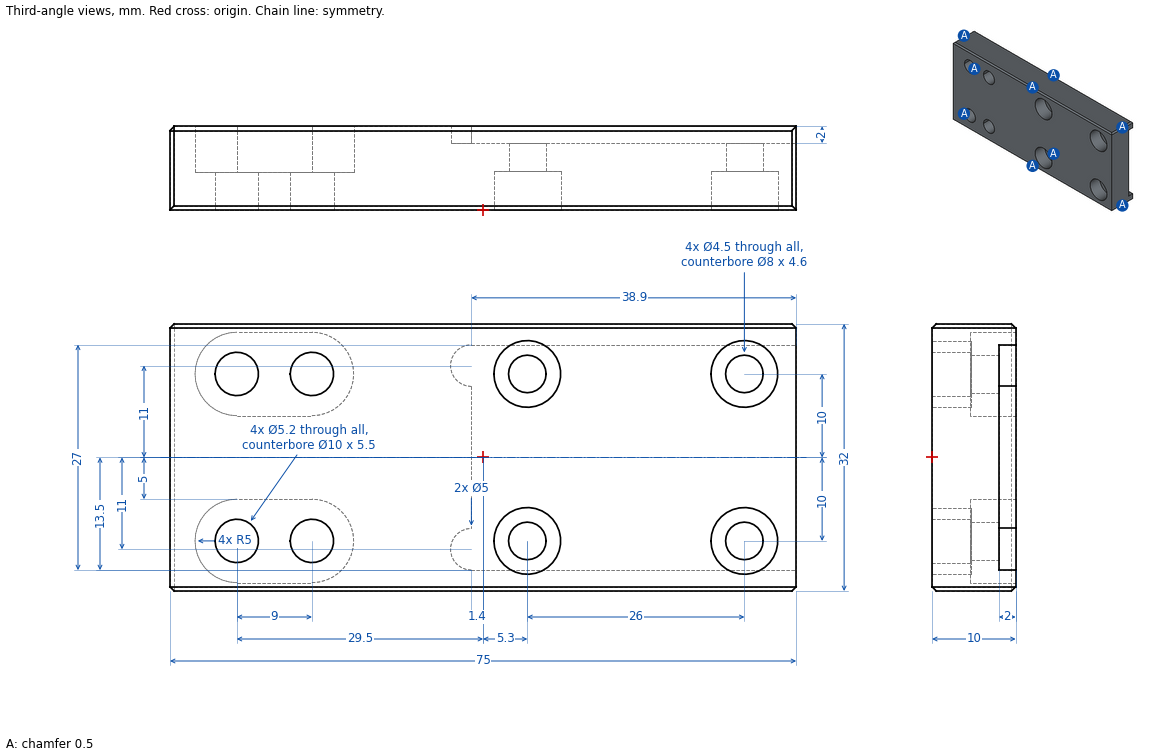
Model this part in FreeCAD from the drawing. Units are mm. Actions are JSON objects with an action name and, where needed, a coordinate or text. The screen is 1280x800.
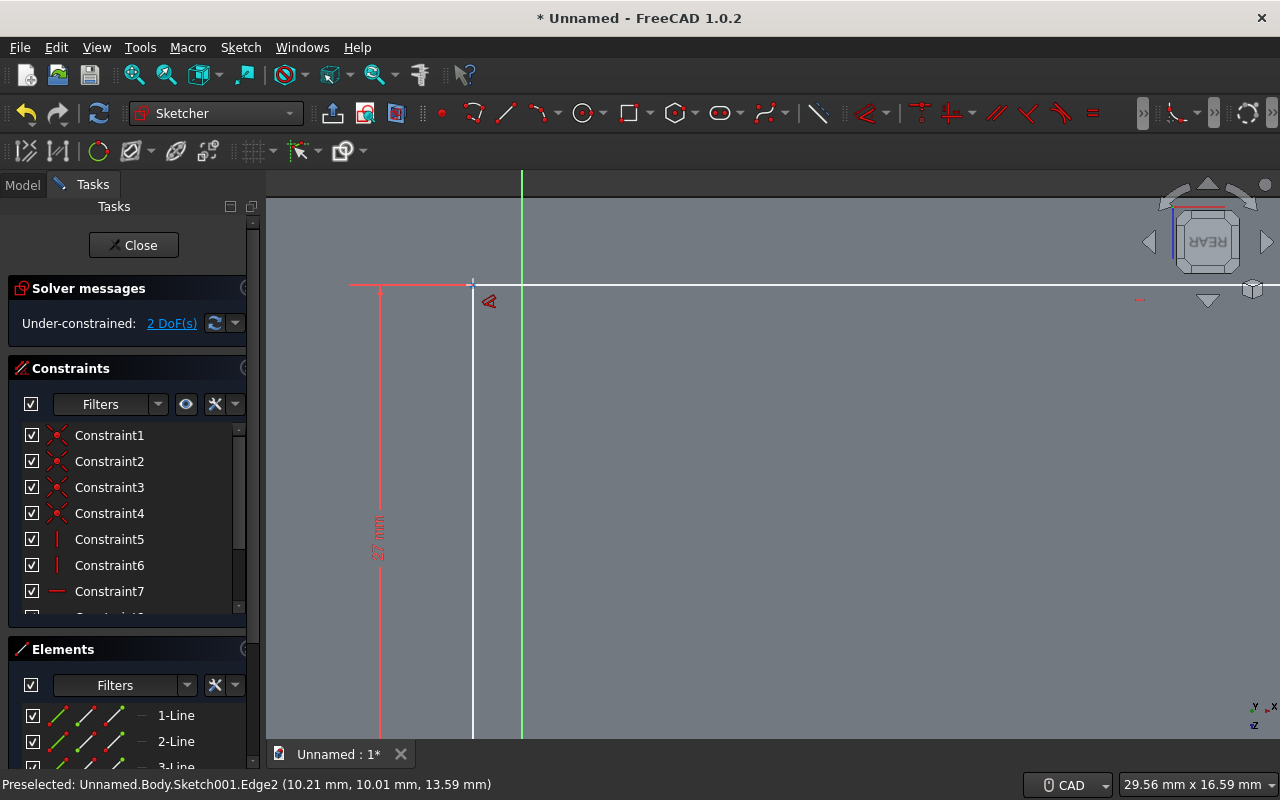
{"action": "left_click", "coordinate": [473, 285]}
{"action": "left_click", "coordinate": [497, 251]}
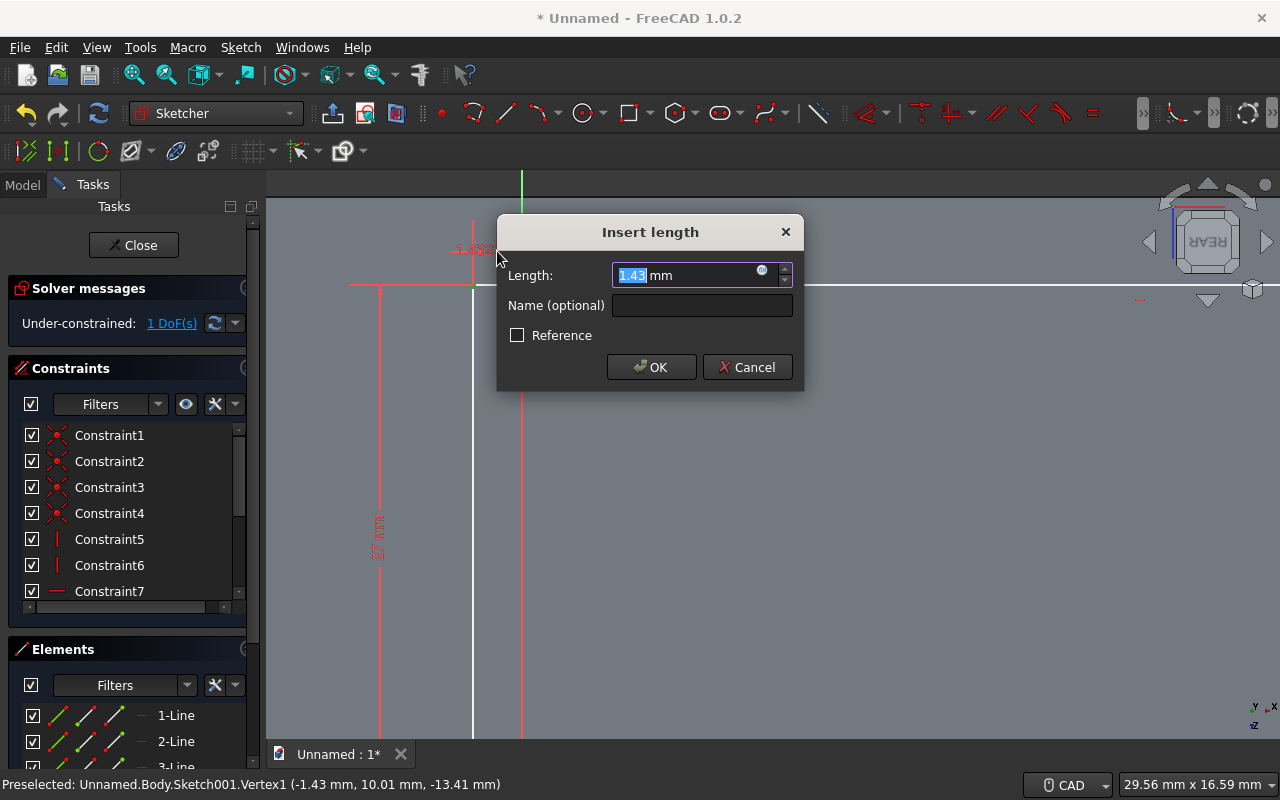
{"action": "type", "text": "1.4"}
{"action": "key", "text": "Return"}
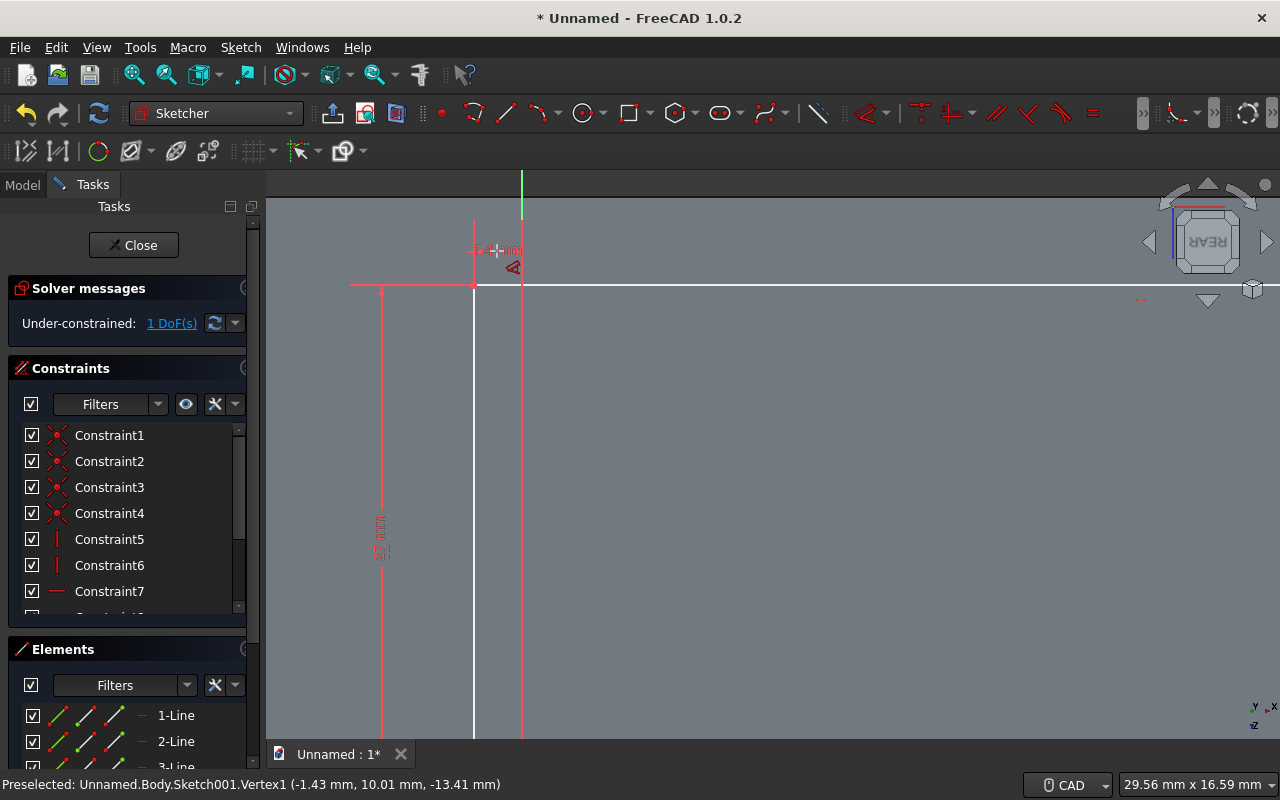
{"action": "left_click", "coordinate": [474, 285]}
{"action": "left_click", "coordinate": [440, 498]}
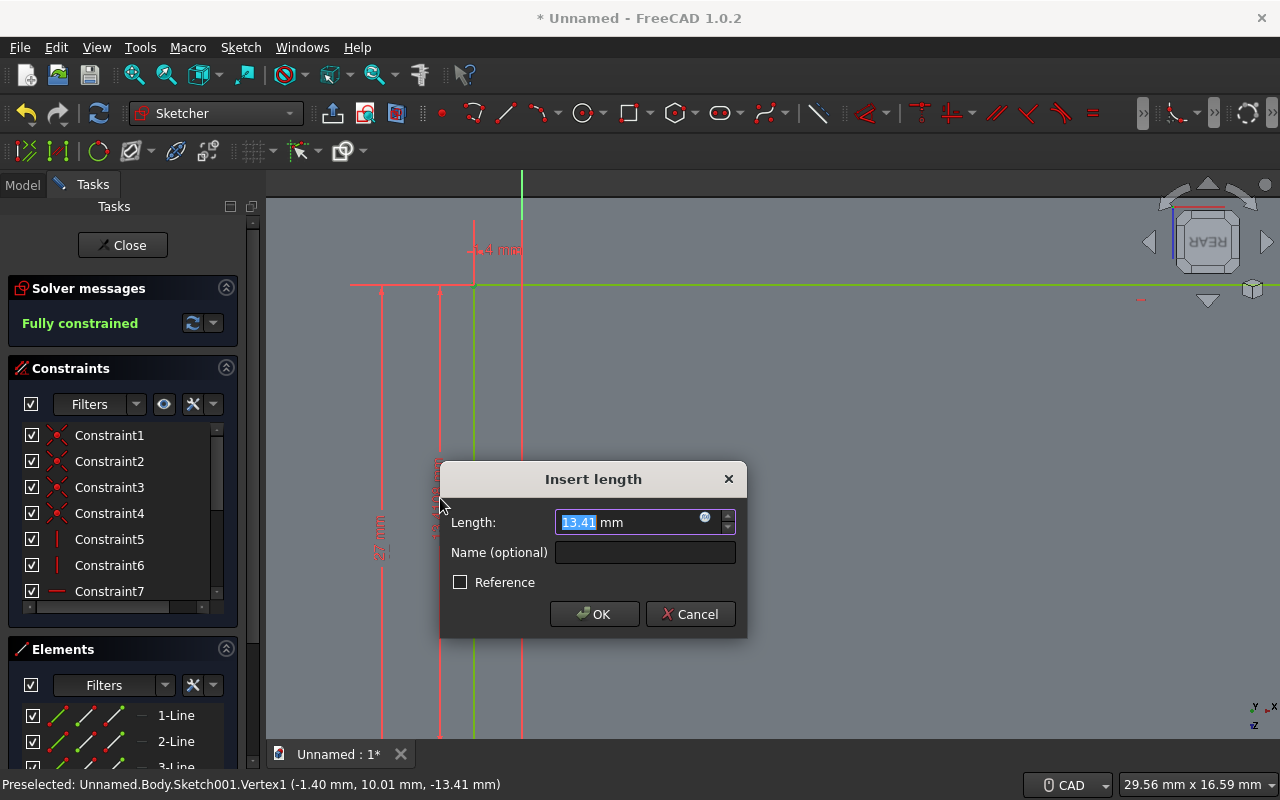
{"action": "type", "text": "13.5"}
{"action": "key", "text": "Return"}
{"action": "key", "text": "Escape"}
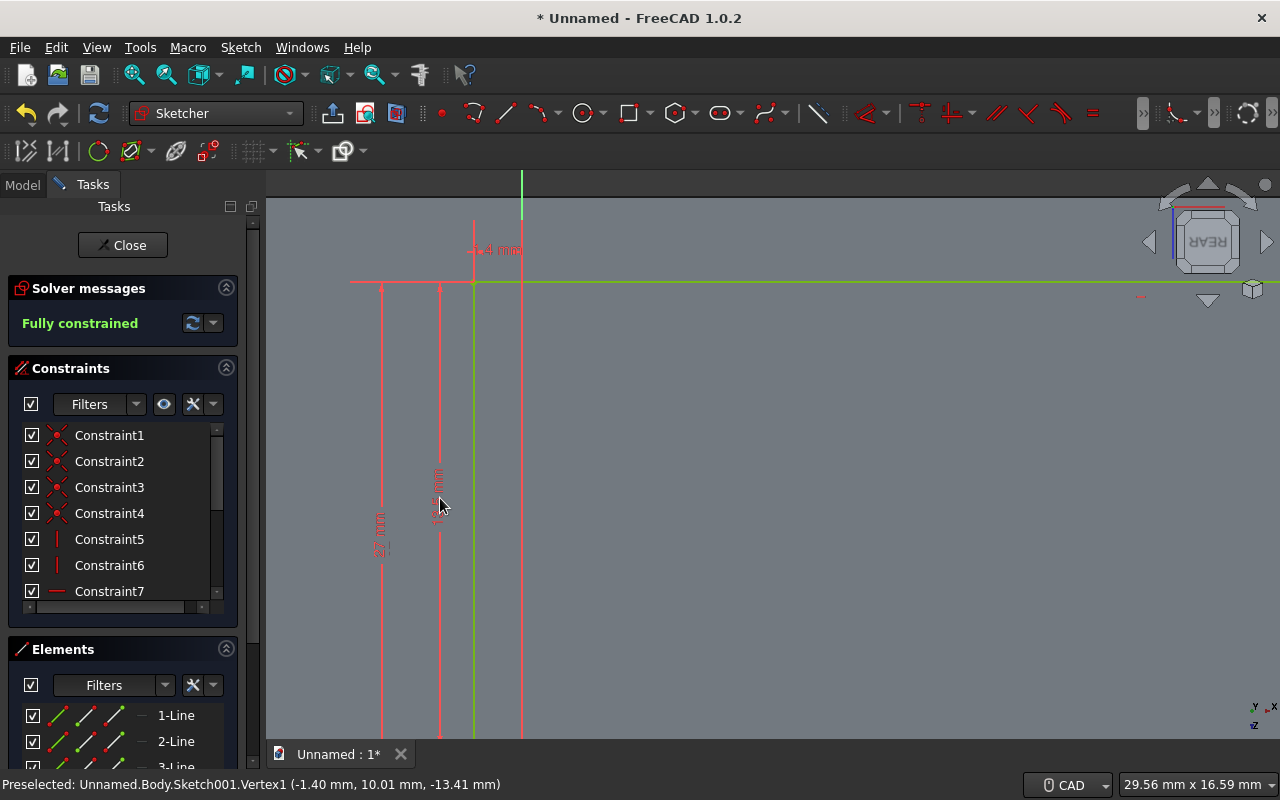
{"action": "left_click", "coordinate": [123, 245]}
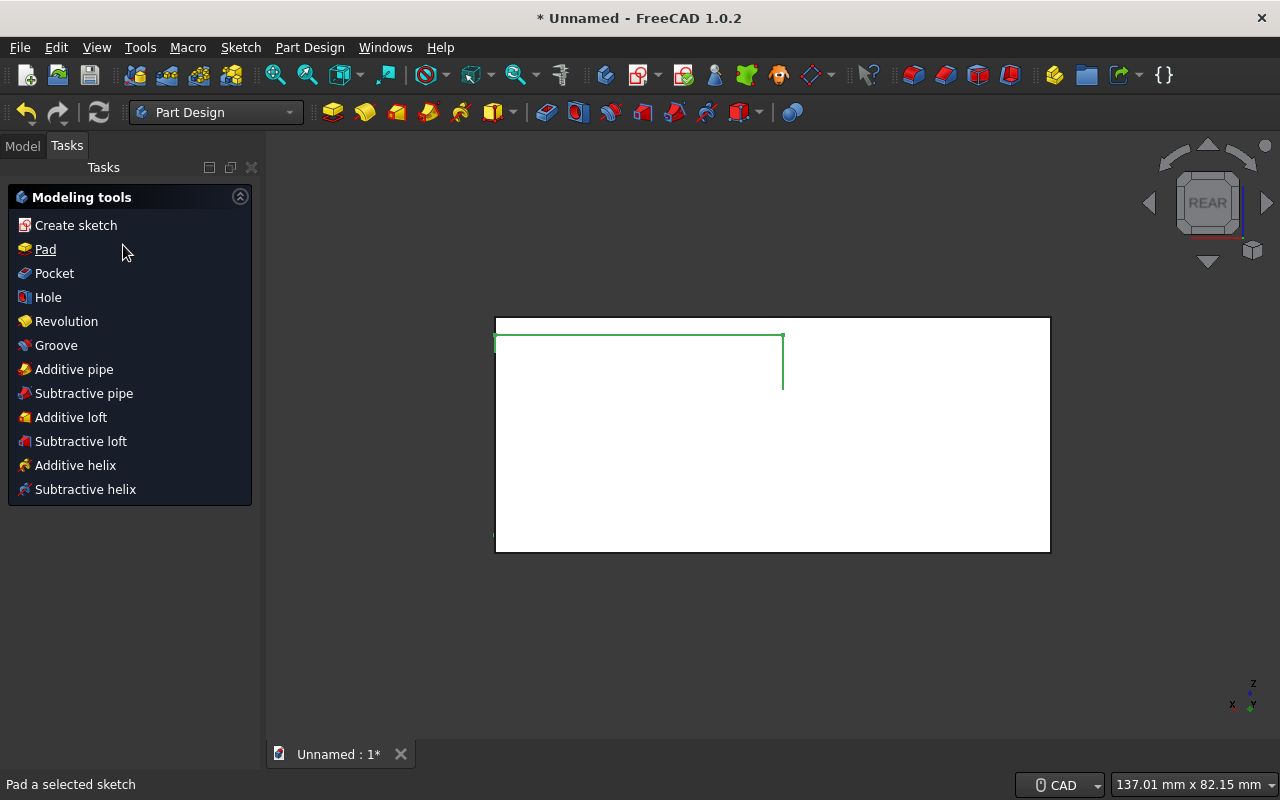
{"action": "left_click", "coordinate": [548, 112]}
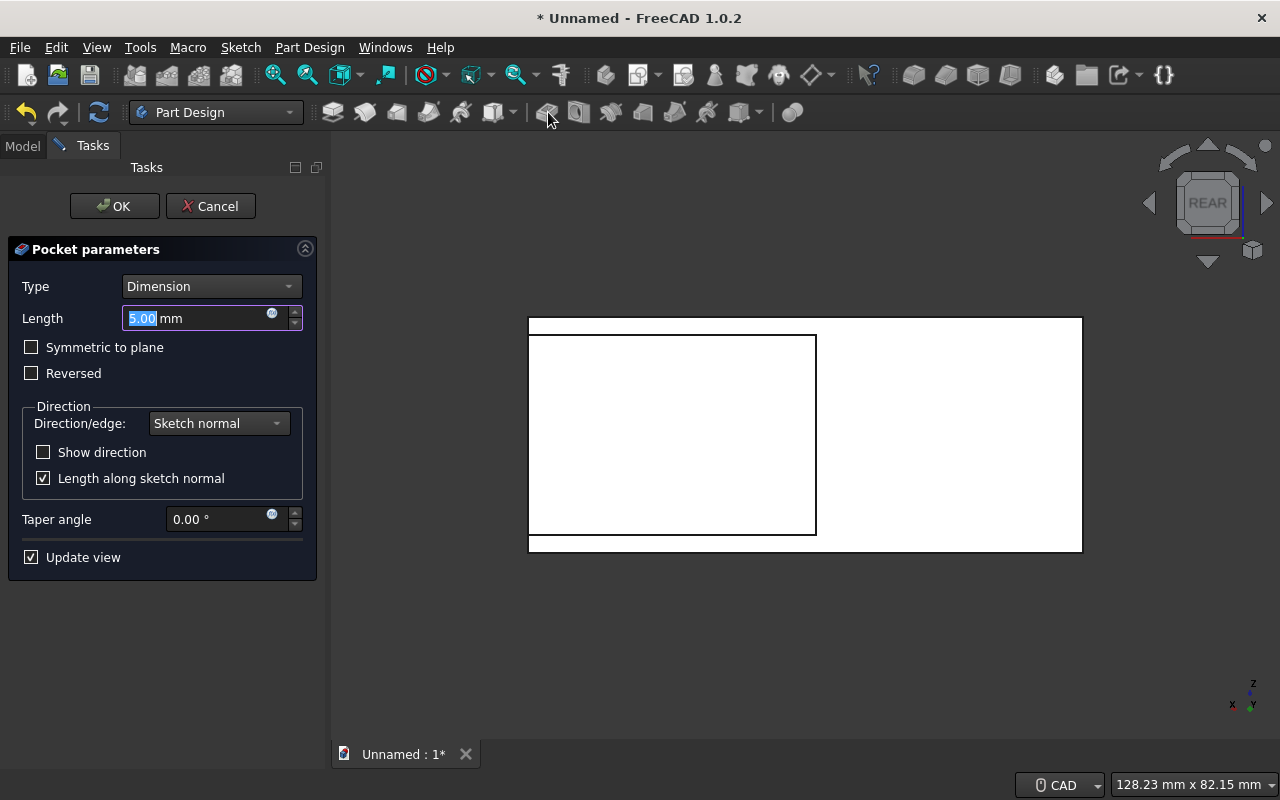
{"action": "type", "text": "2"}
{"action": "key", "text": "Tab"}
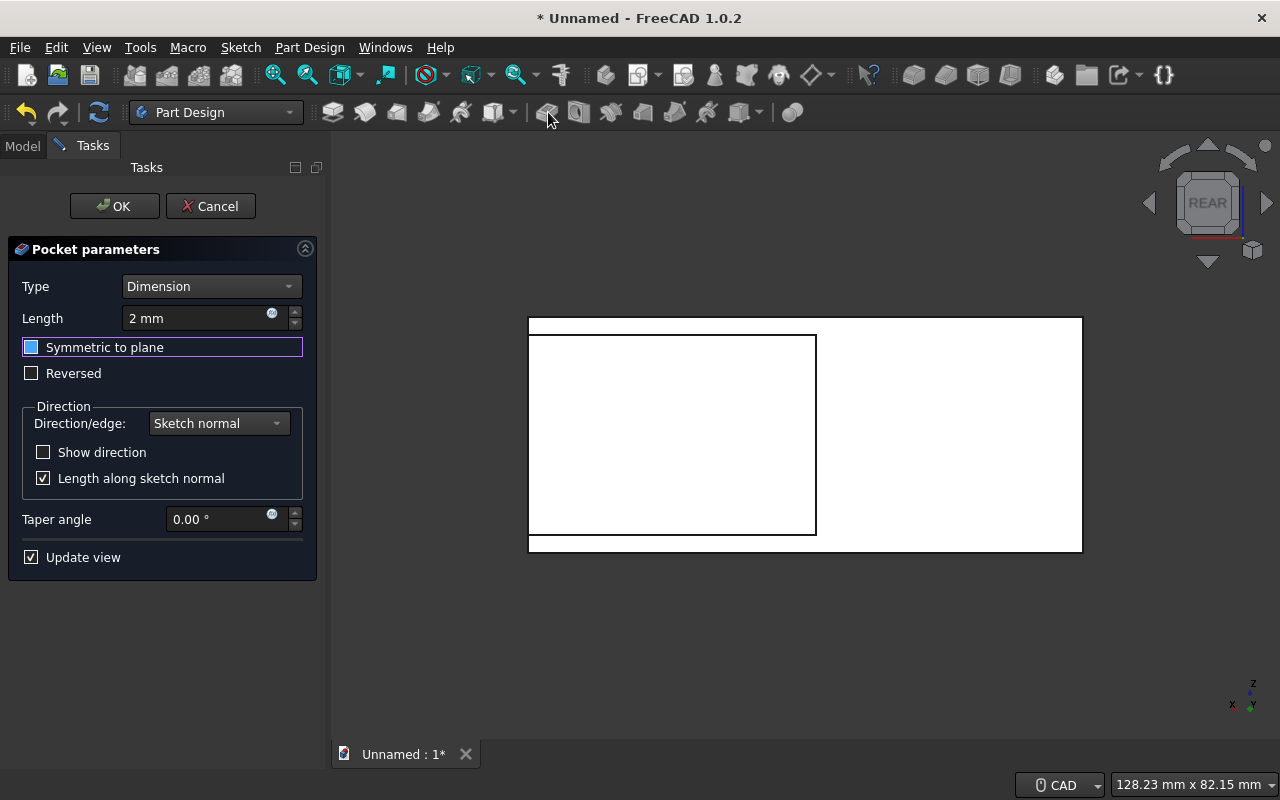
{"action": "left_click", "coordinate": [115, 206]}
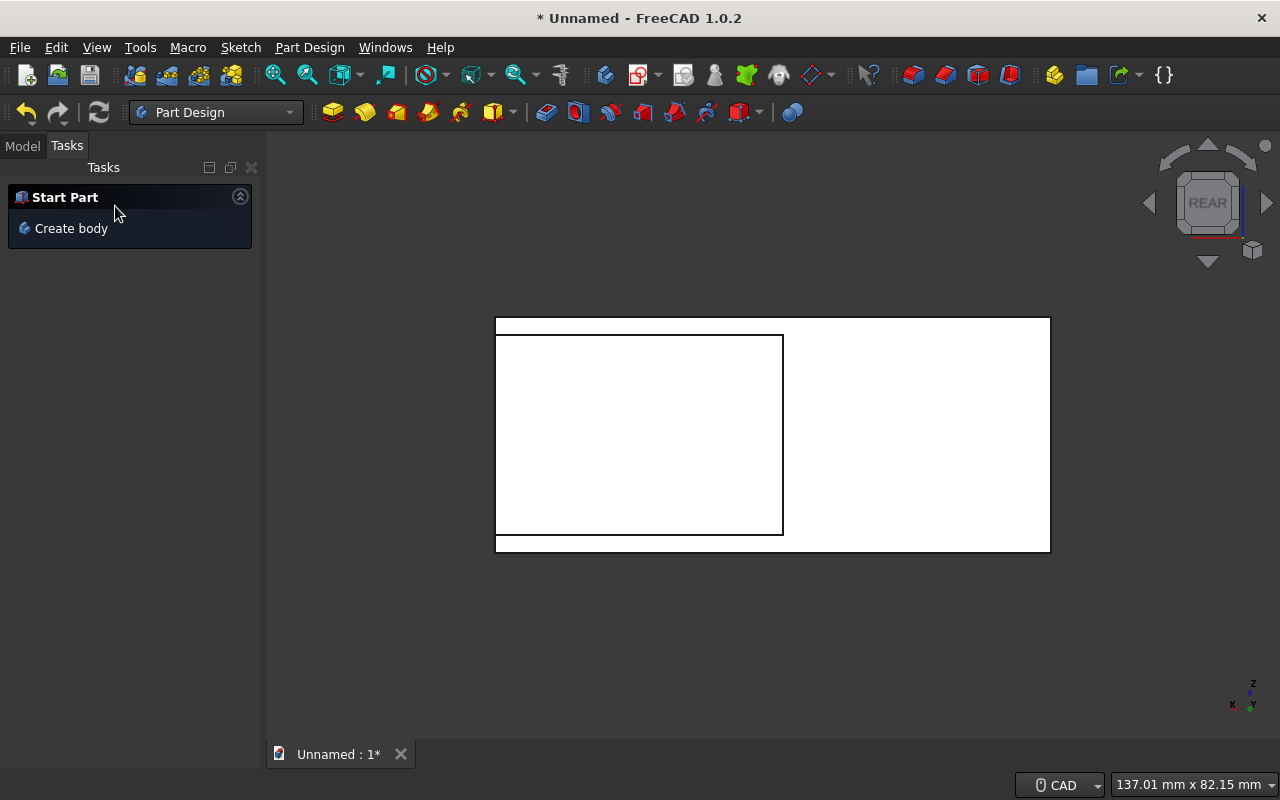
{"action": "left_click", "coordinate": [638, 76]}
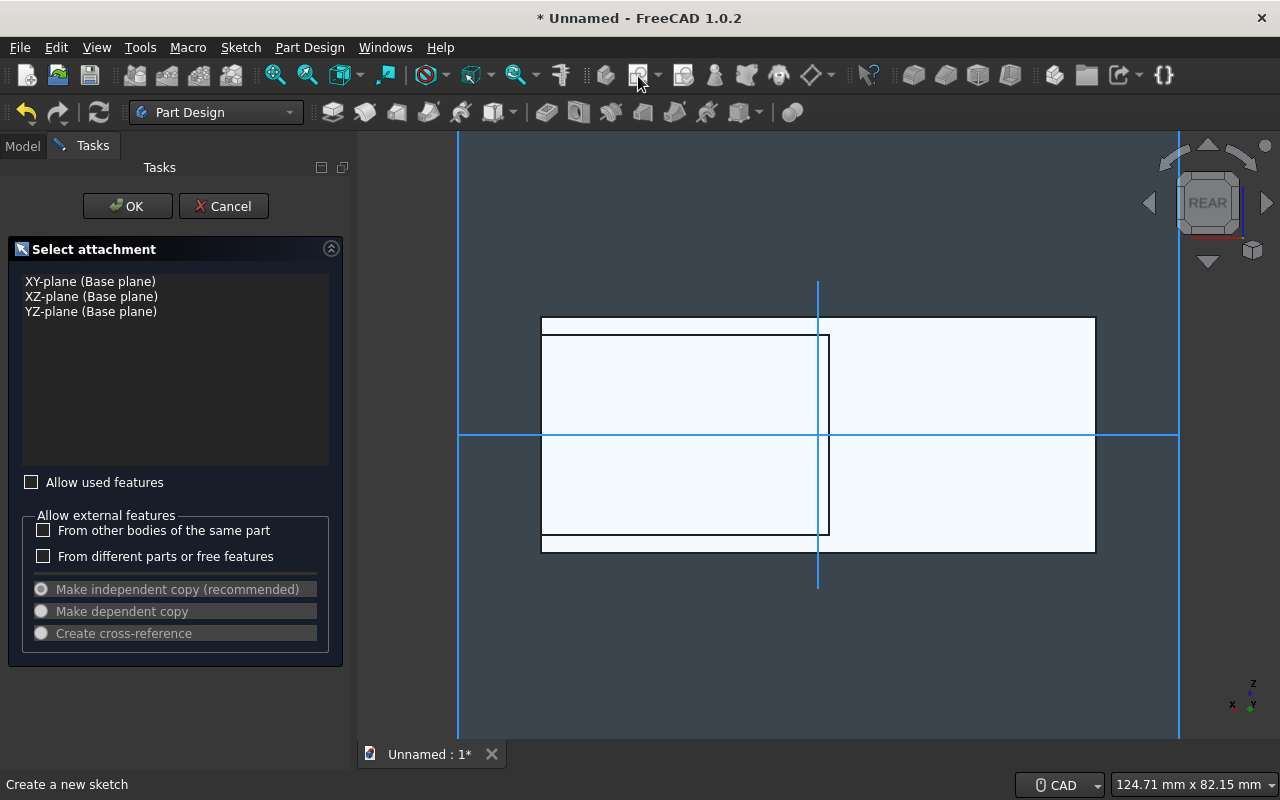
{"action": "left_click", "coordinate": [82, 296]}